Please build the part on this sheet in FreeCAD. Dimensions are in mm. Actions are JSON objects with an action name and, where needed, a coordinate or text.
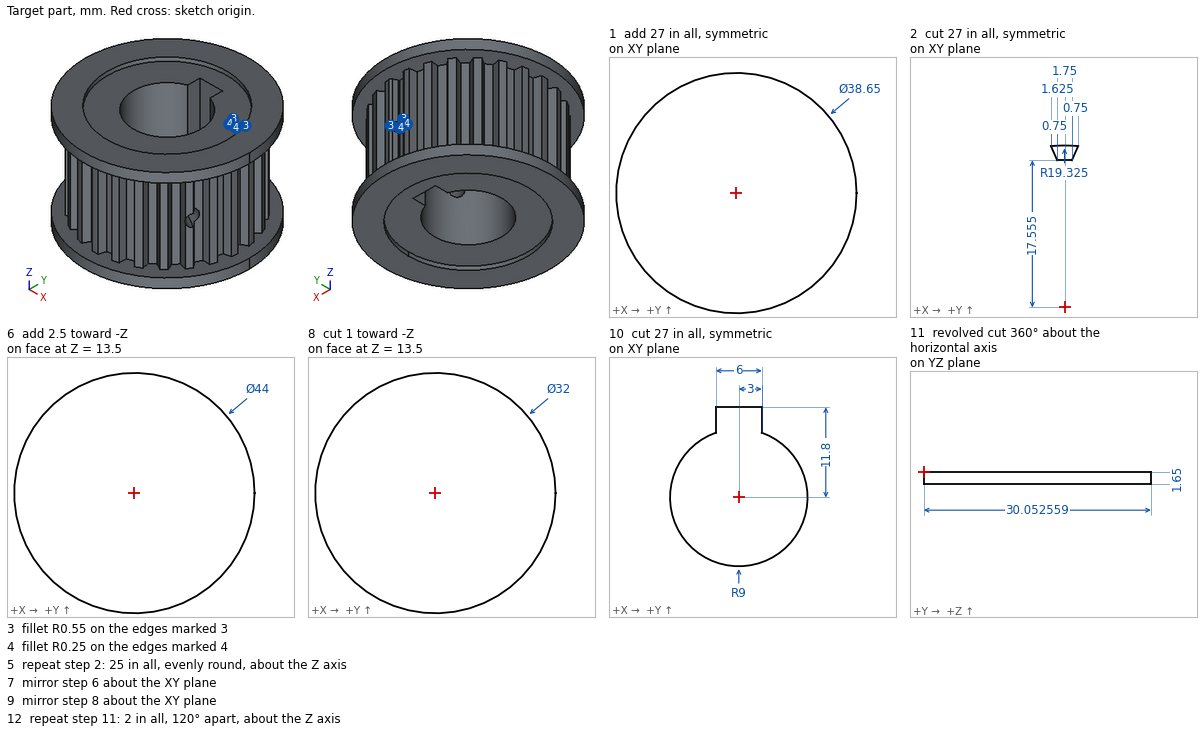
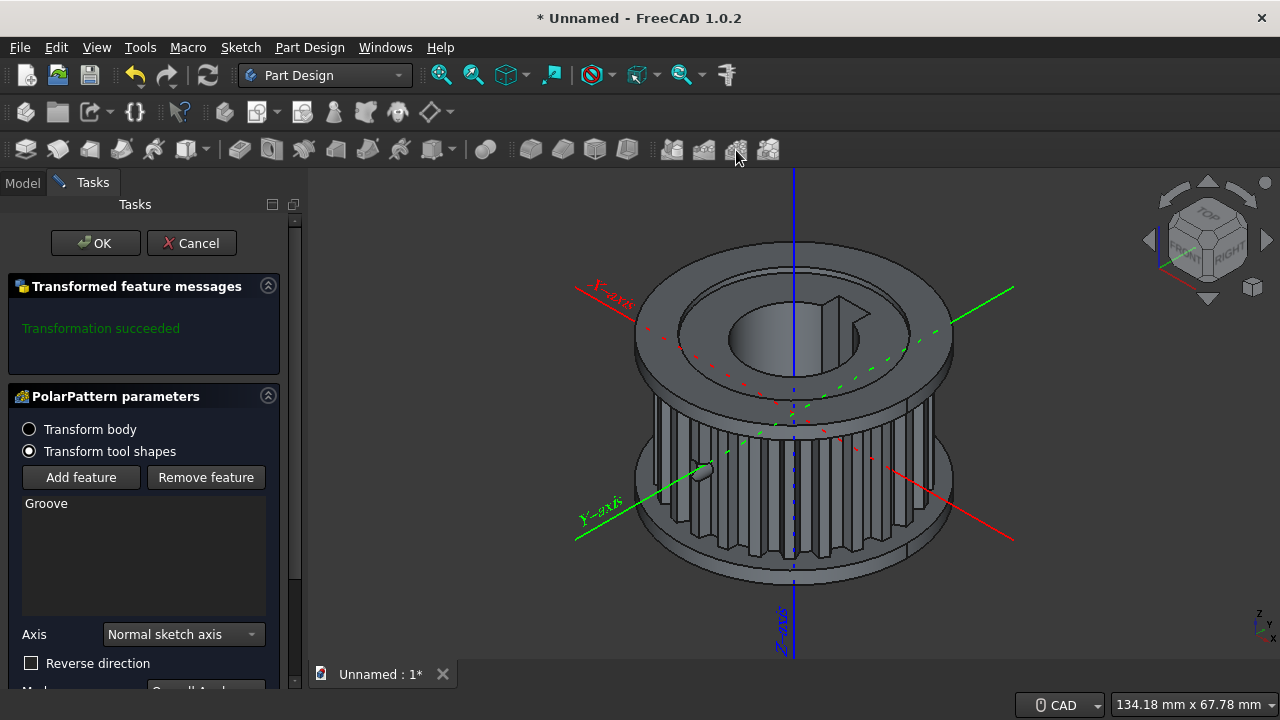
{"action": "left_click", "coordinate": [184, 634]}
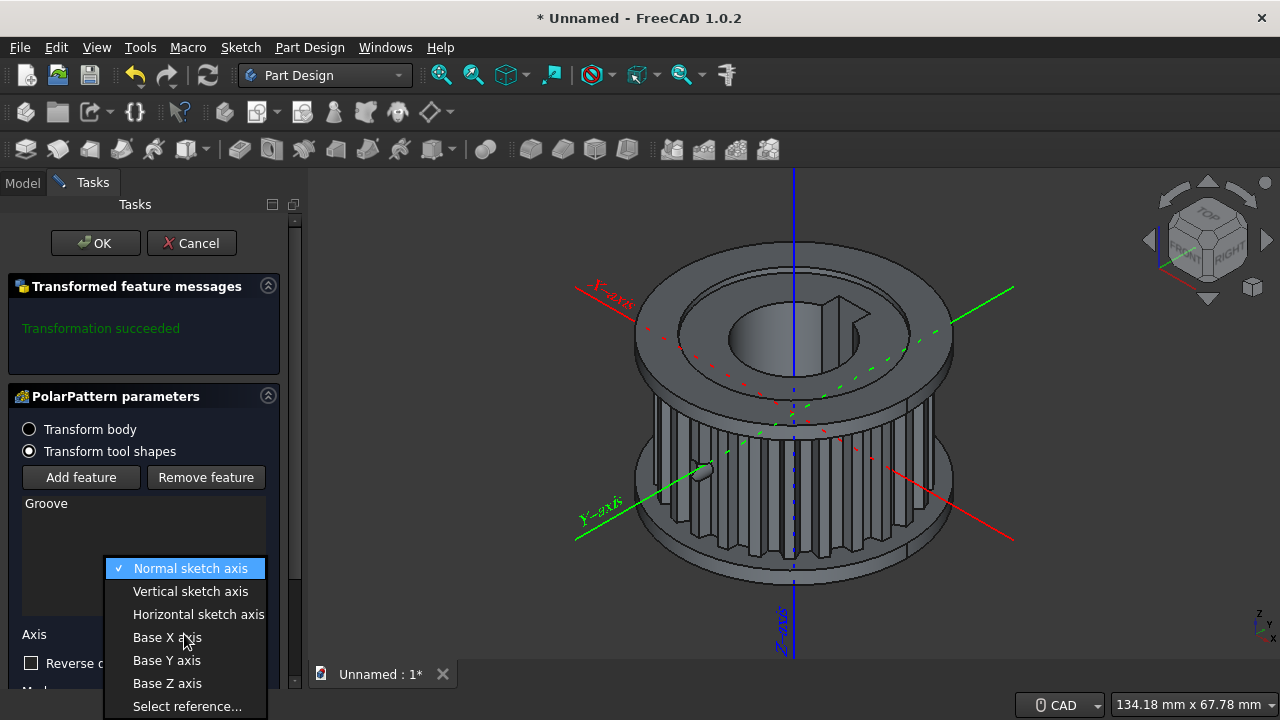
{"action": "left_click", "coordinate": [184, 684]}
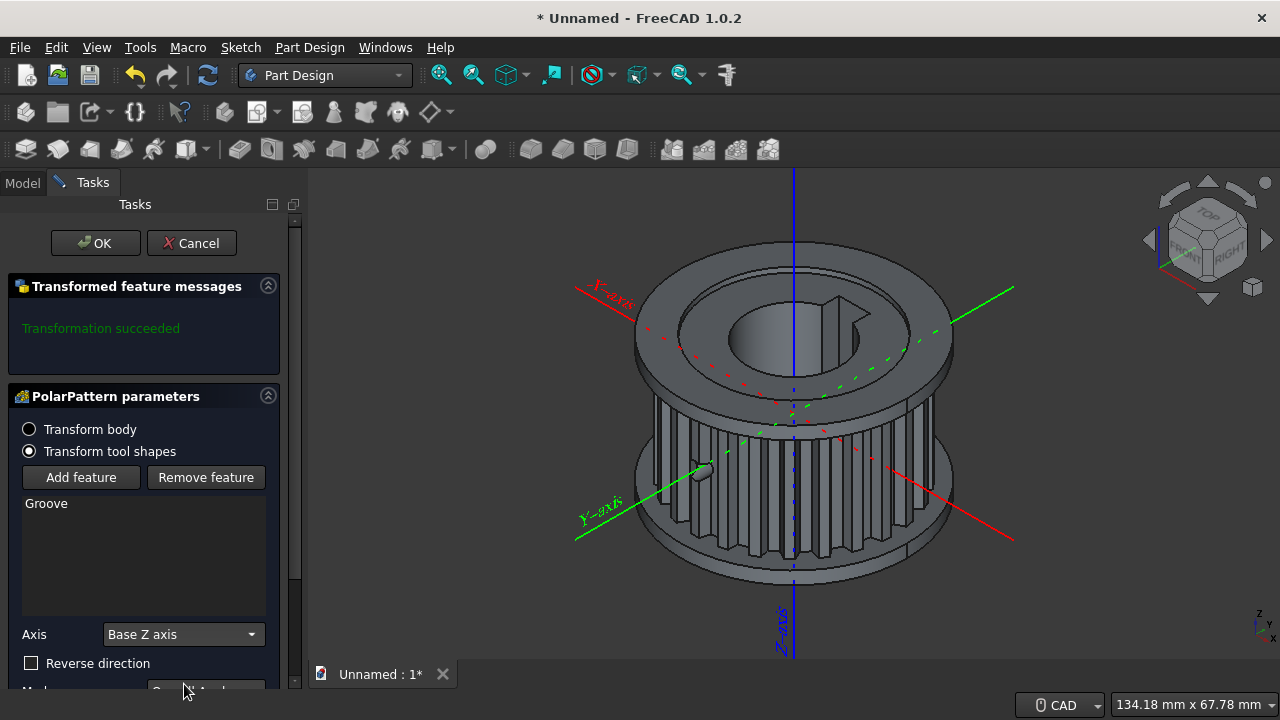
{"action": "scroll", "coordinate": [295, 451], "scroll_direction": "down", "scroll_amount": 2}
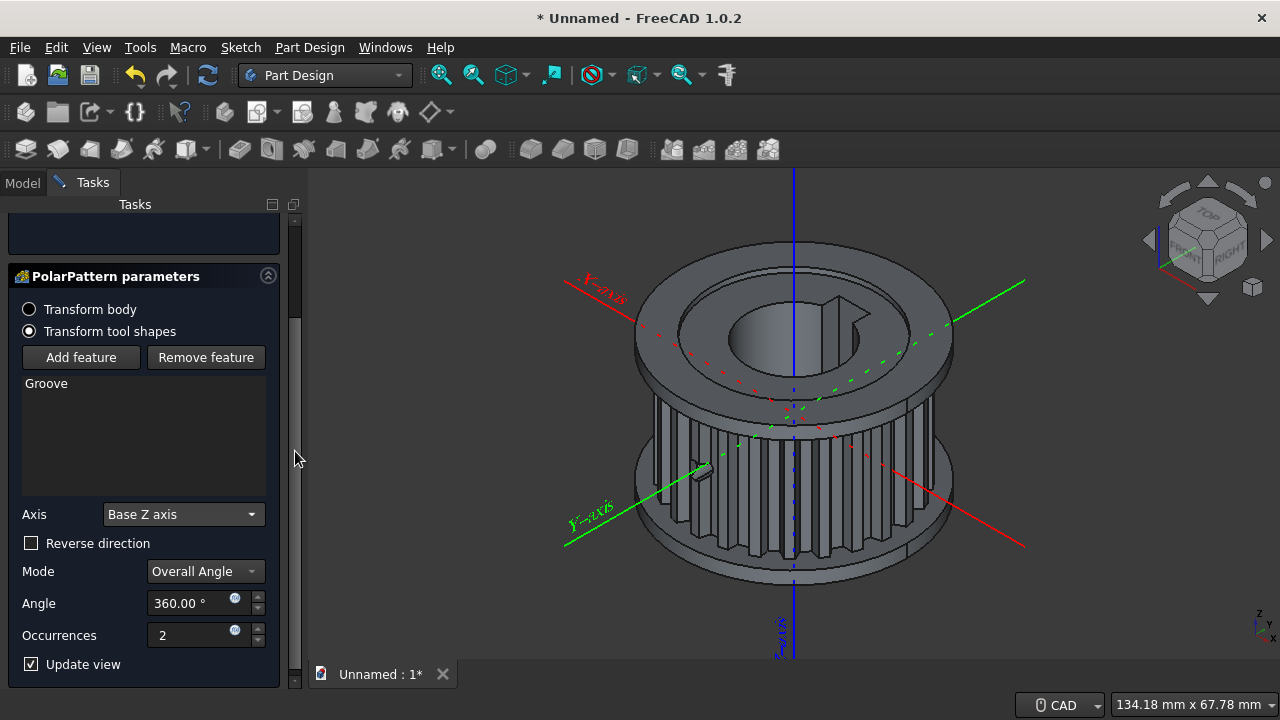
{"action": "left_click", "coordinate": [206, 572]}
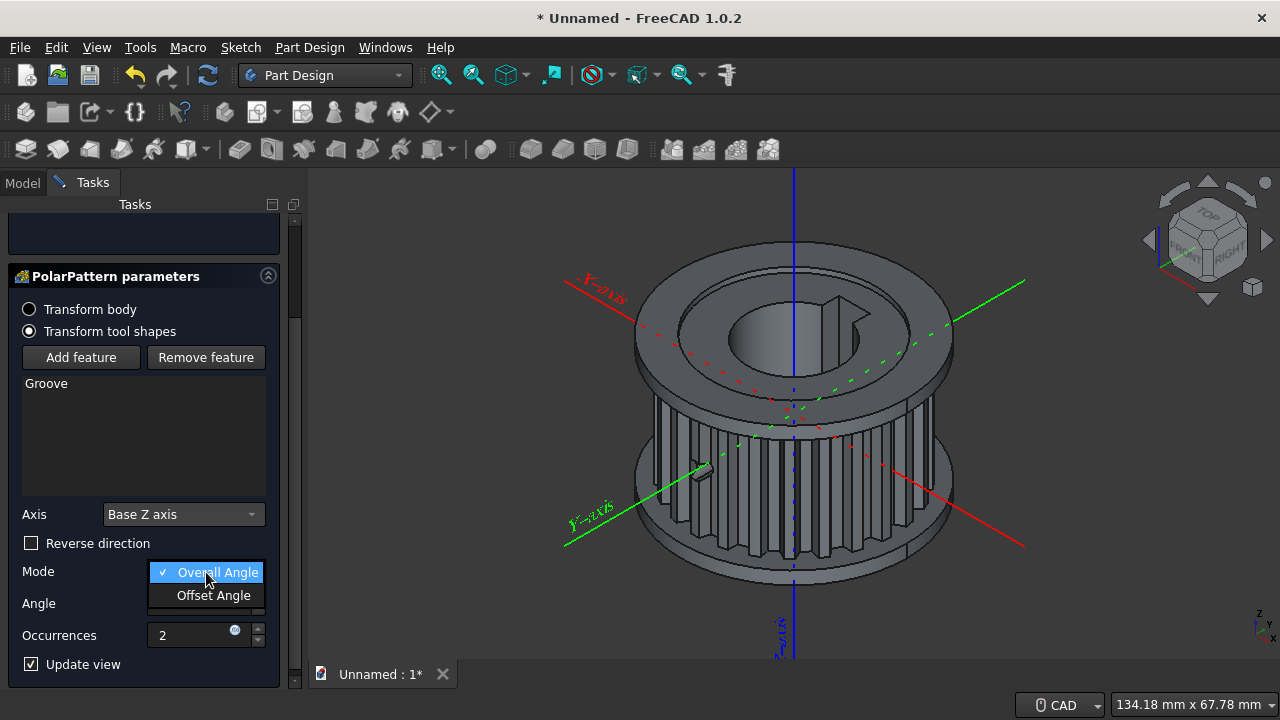
{"action": "left_click", "coordinate": [206, 596]}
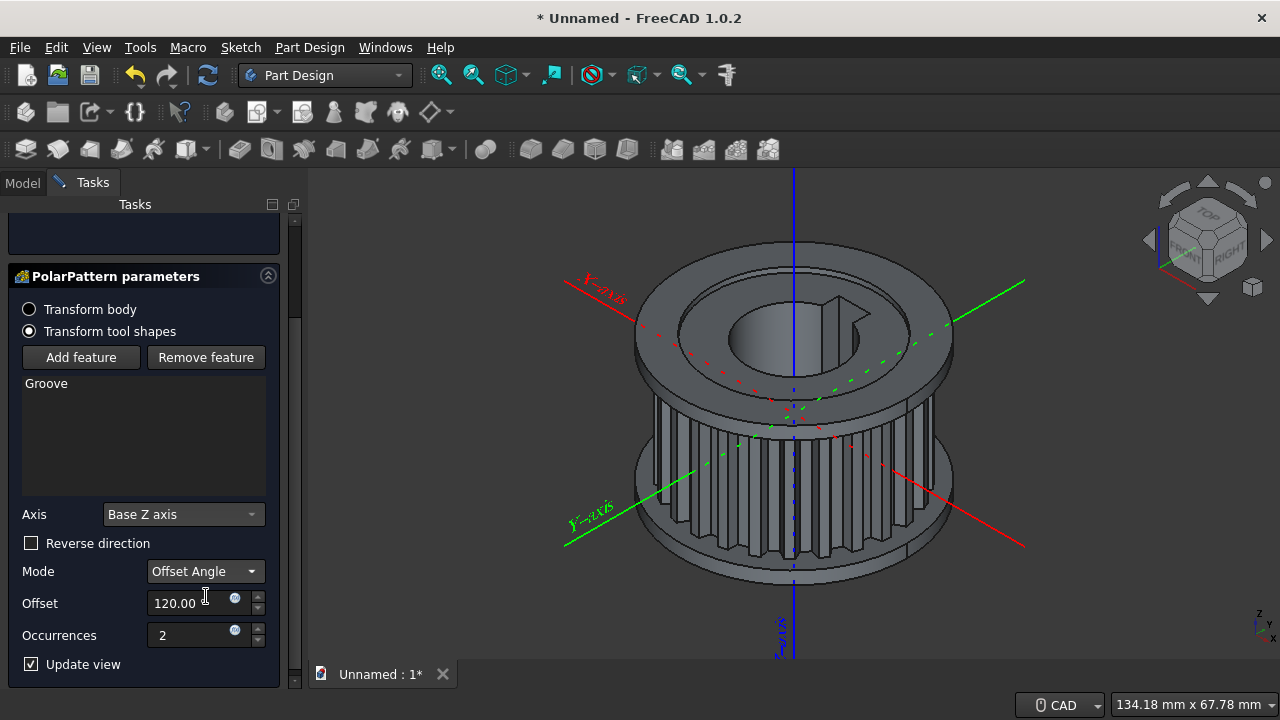
{"action": "triple_click", "coordinate": [198, 603]}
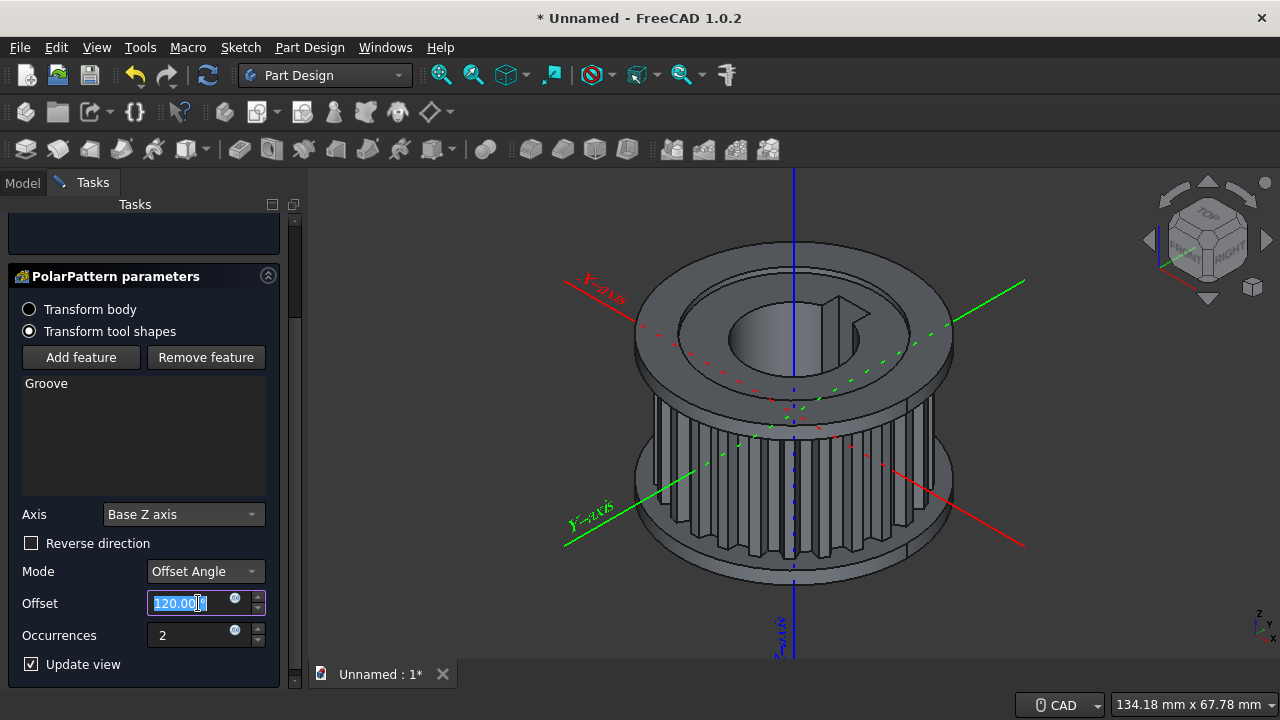
{"action": "type", "text": "120"}
{"action": "key", "text": "Tab"}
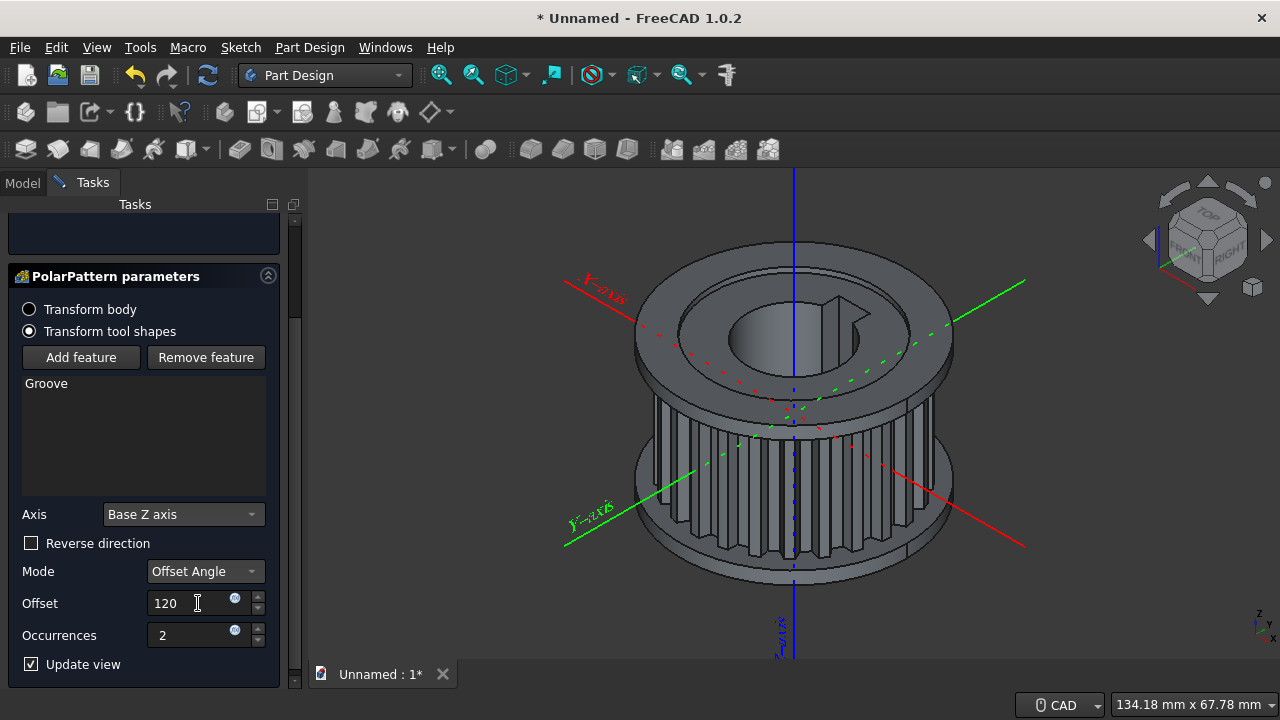
{"action": "triple_click", "coordinate": [198, 635]}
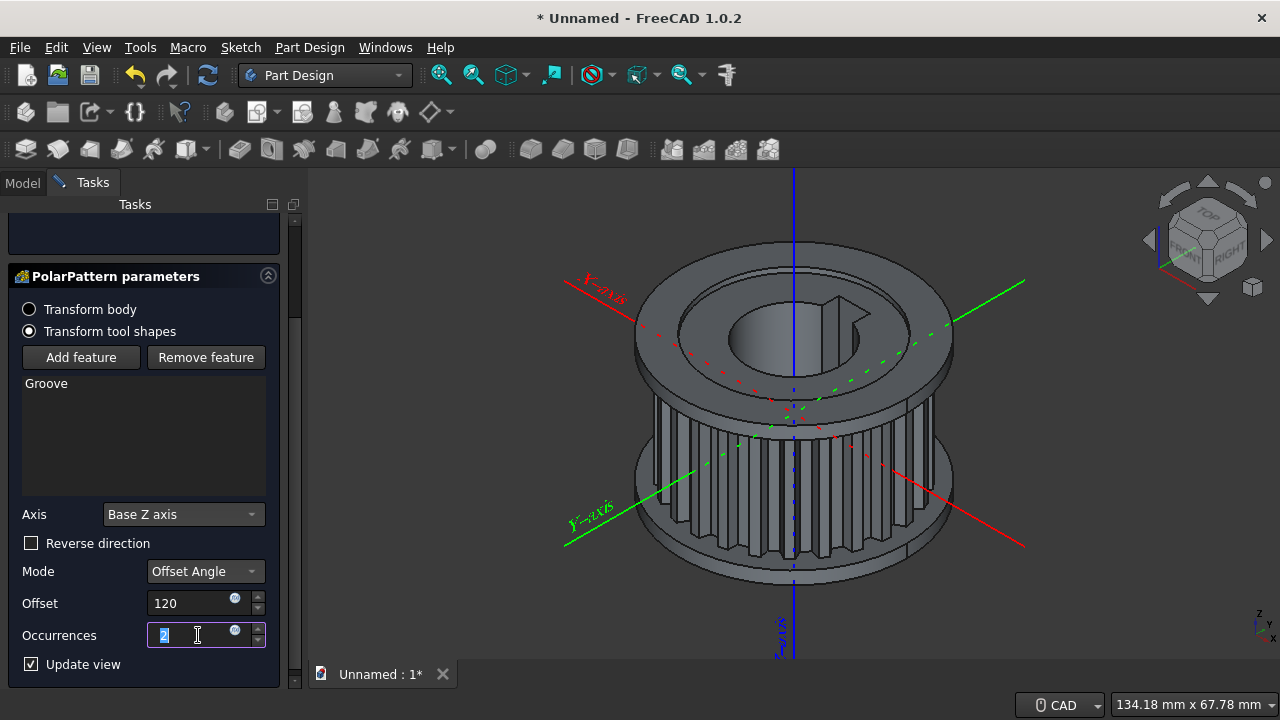
{"action": "type", "text": "2"}
{"action": "key", "text": "Tab"}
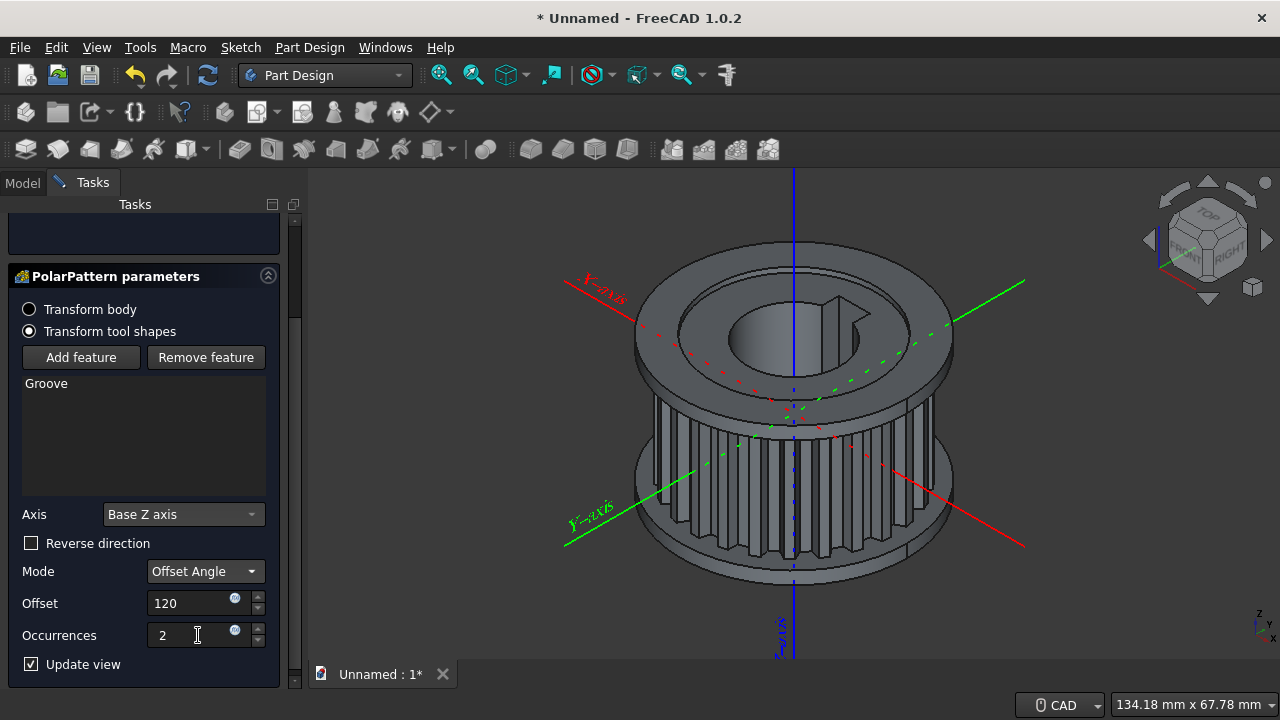
{"action": "left_click", "coordinate": [30, 543]}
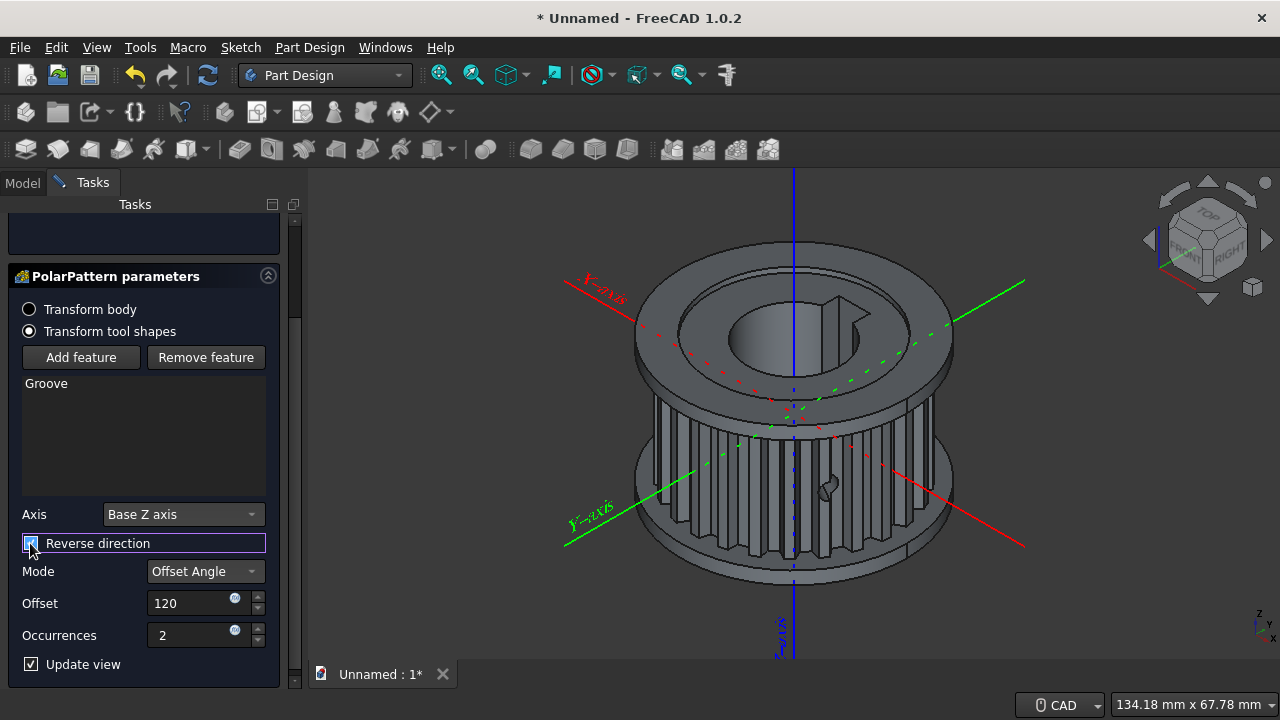
{"action": "scroll", "coordinate": [295, 451], "scroll_direction": "up", "scroll_amount": 3}